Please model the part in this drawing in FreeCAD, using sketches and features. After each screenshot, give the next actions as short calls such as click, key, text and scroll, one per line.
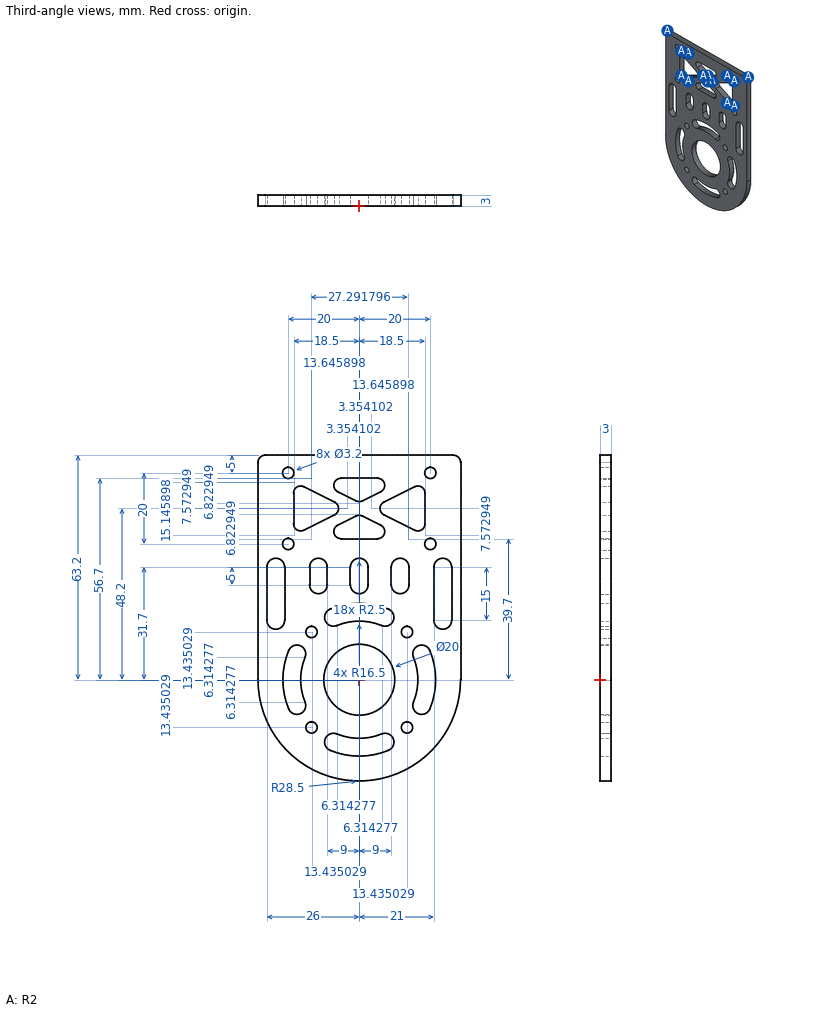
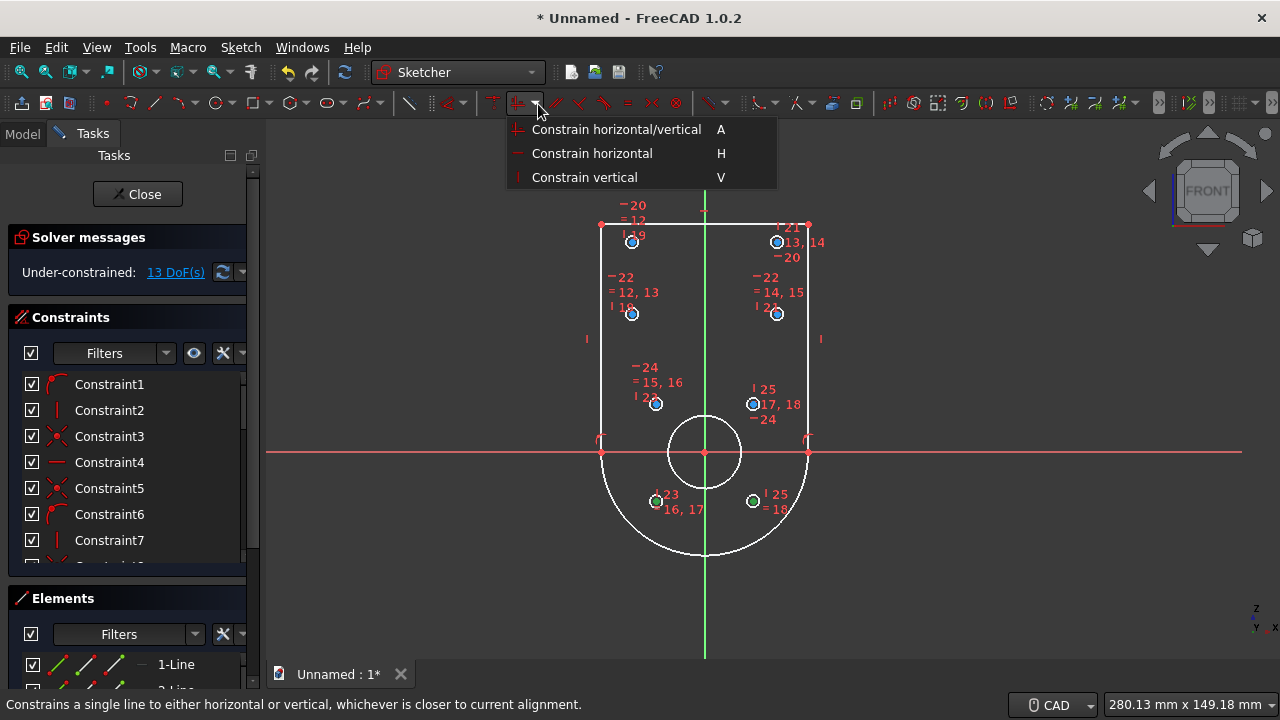
click(642, 153)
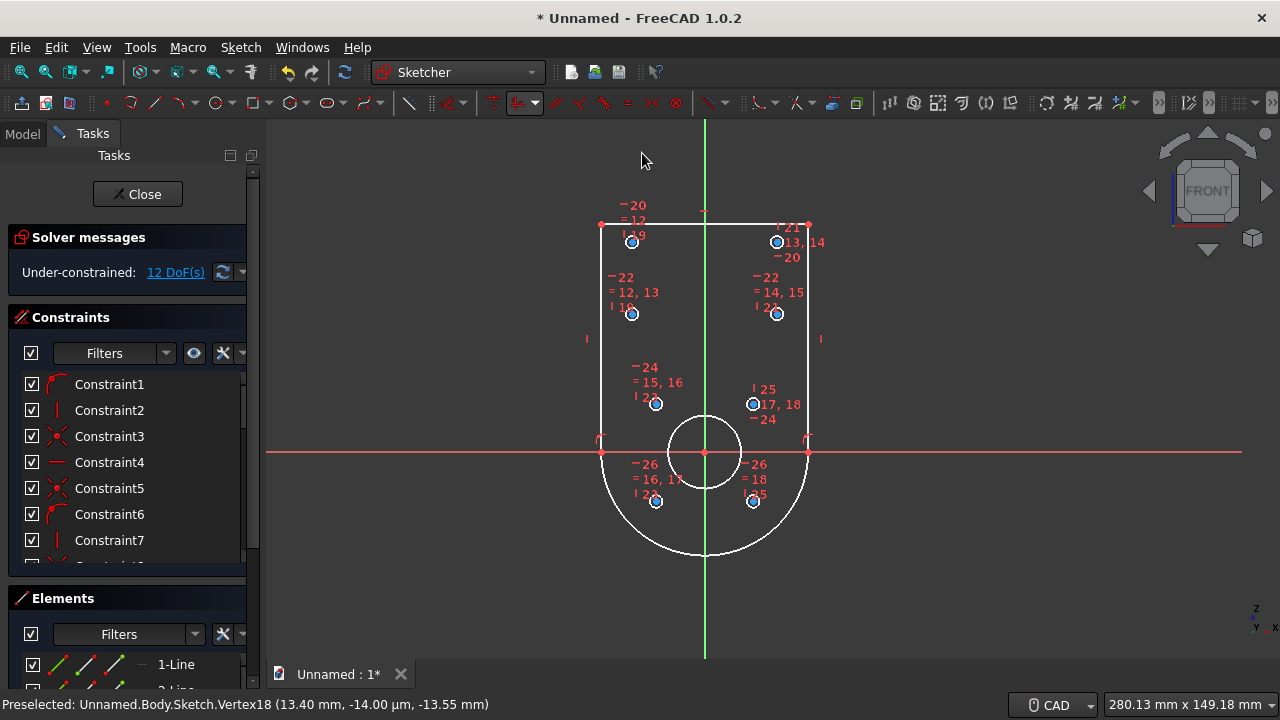
key(d)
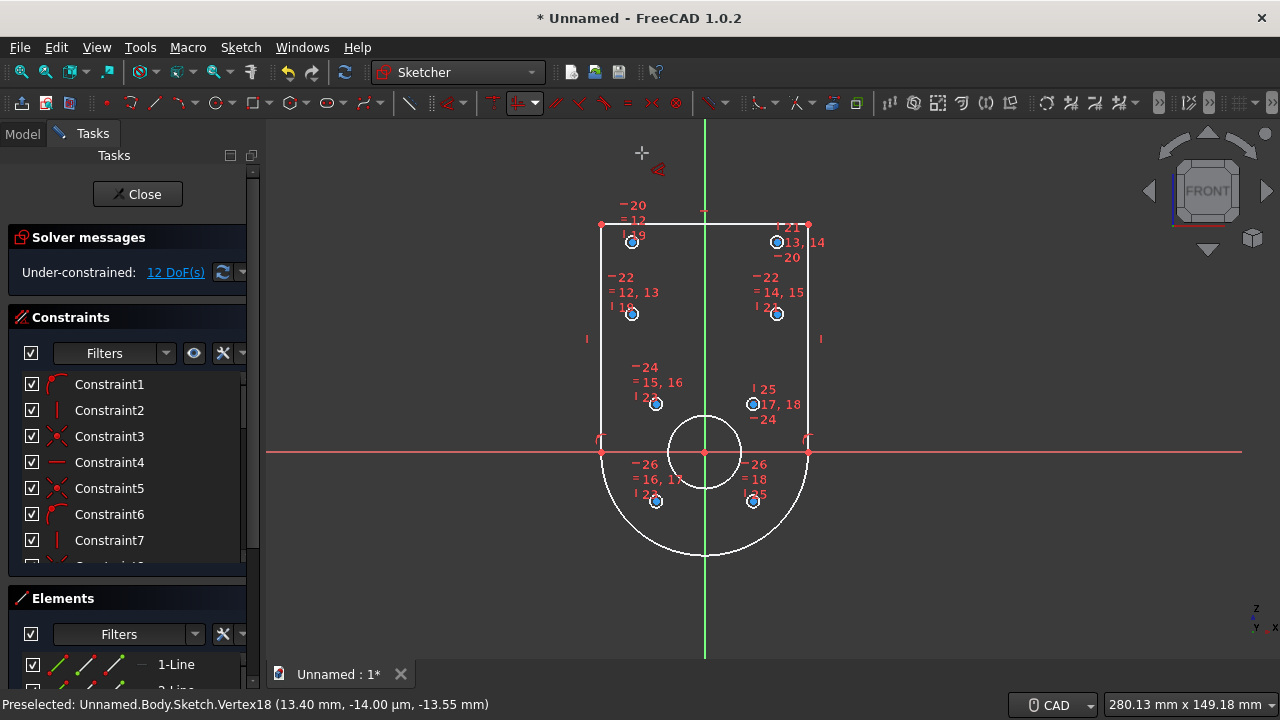
click(644, 536)
click(625, 562)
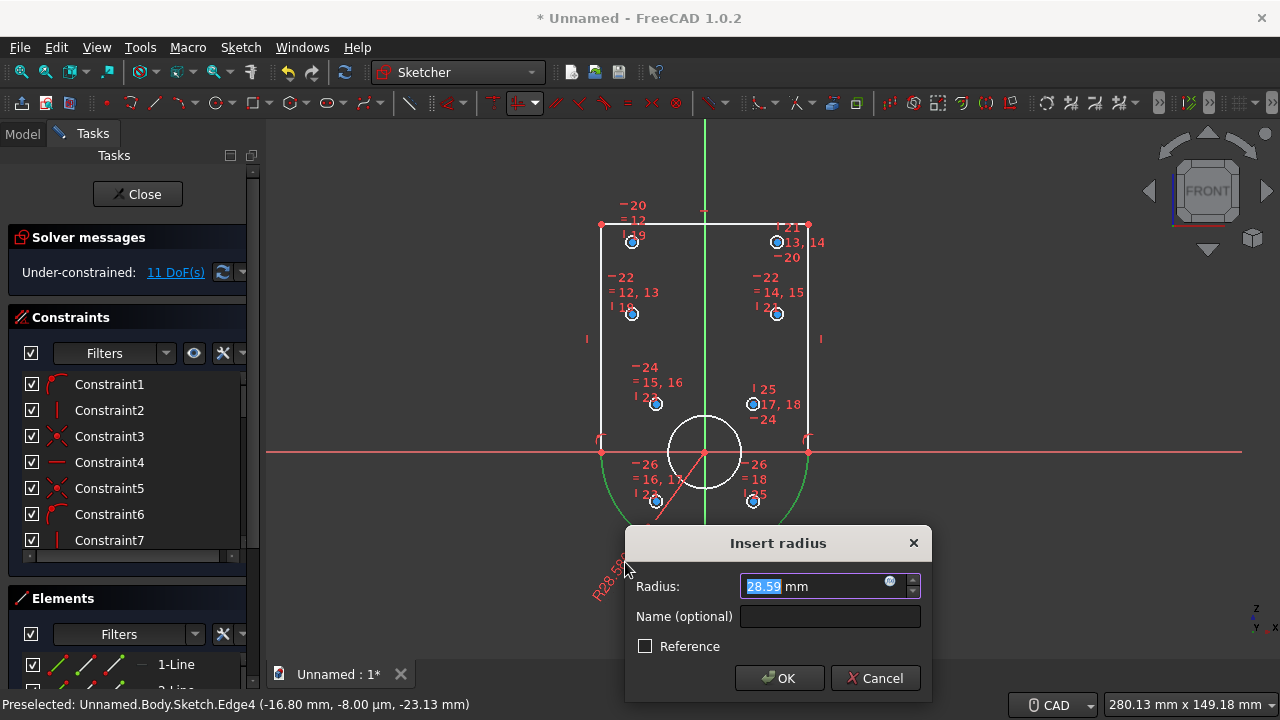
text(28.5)
key(Return)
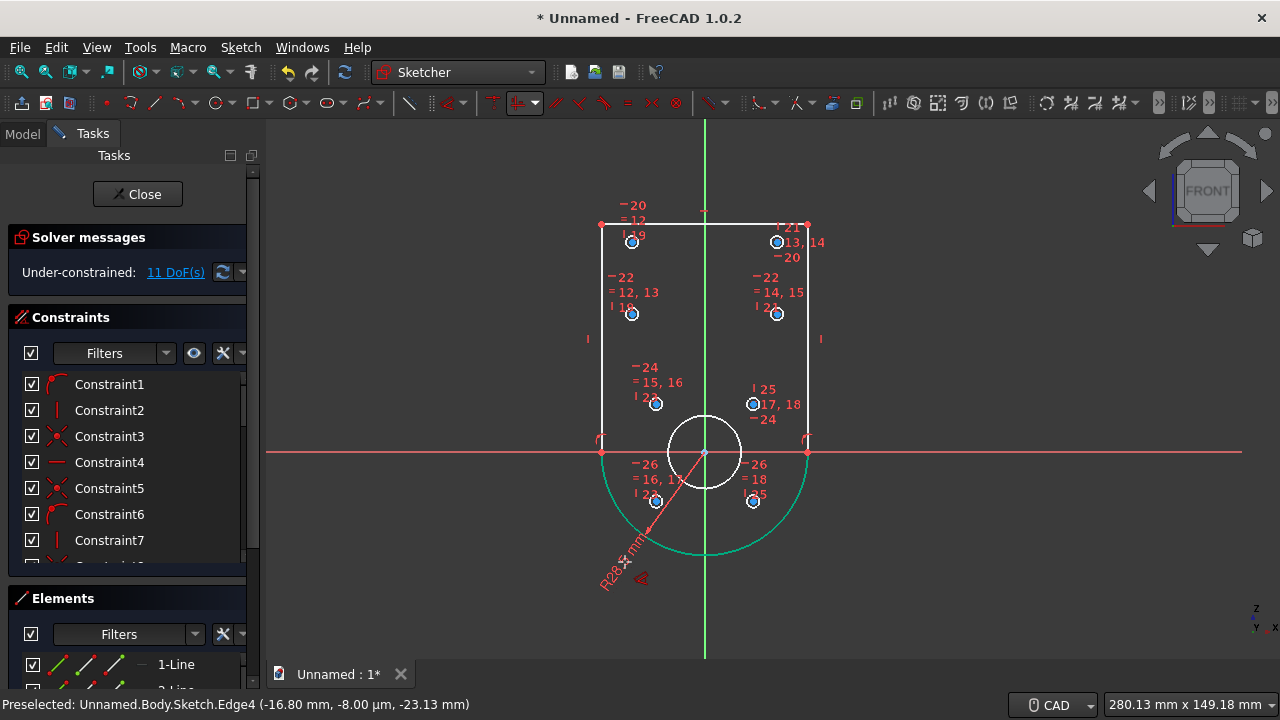
scroll(632, 248, up, 7)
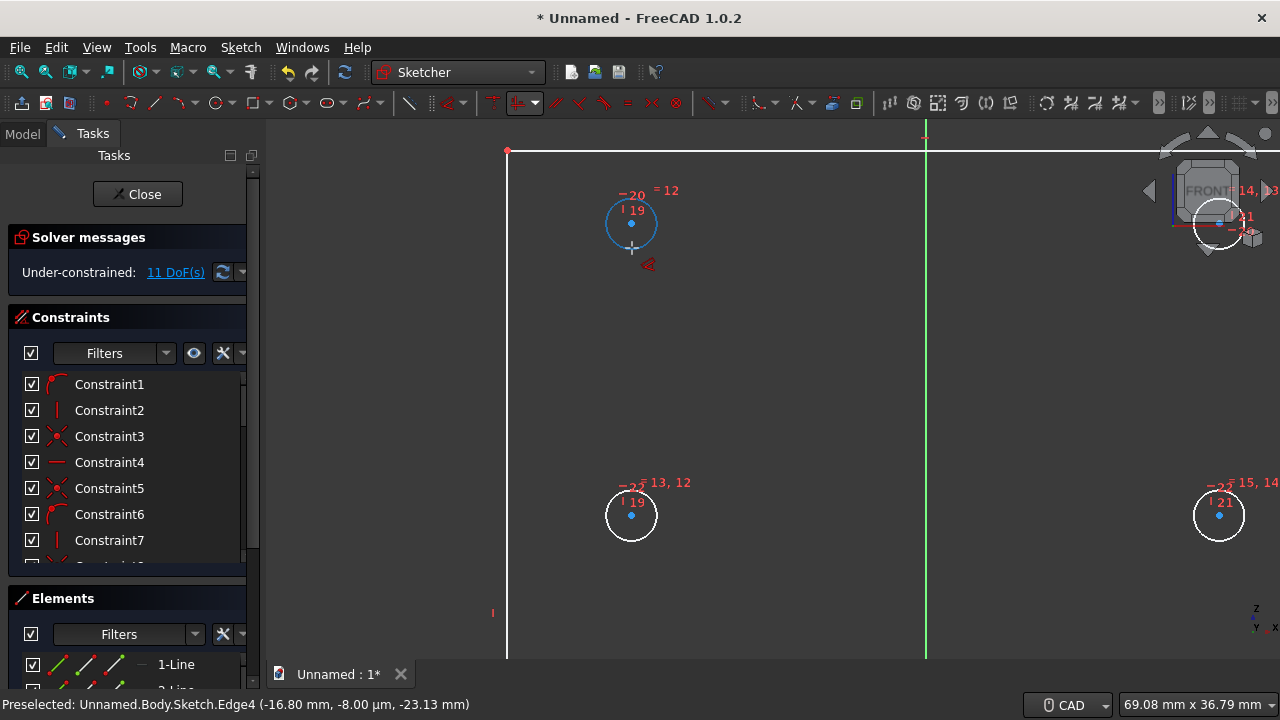
click(631, 249)
click(630, 281)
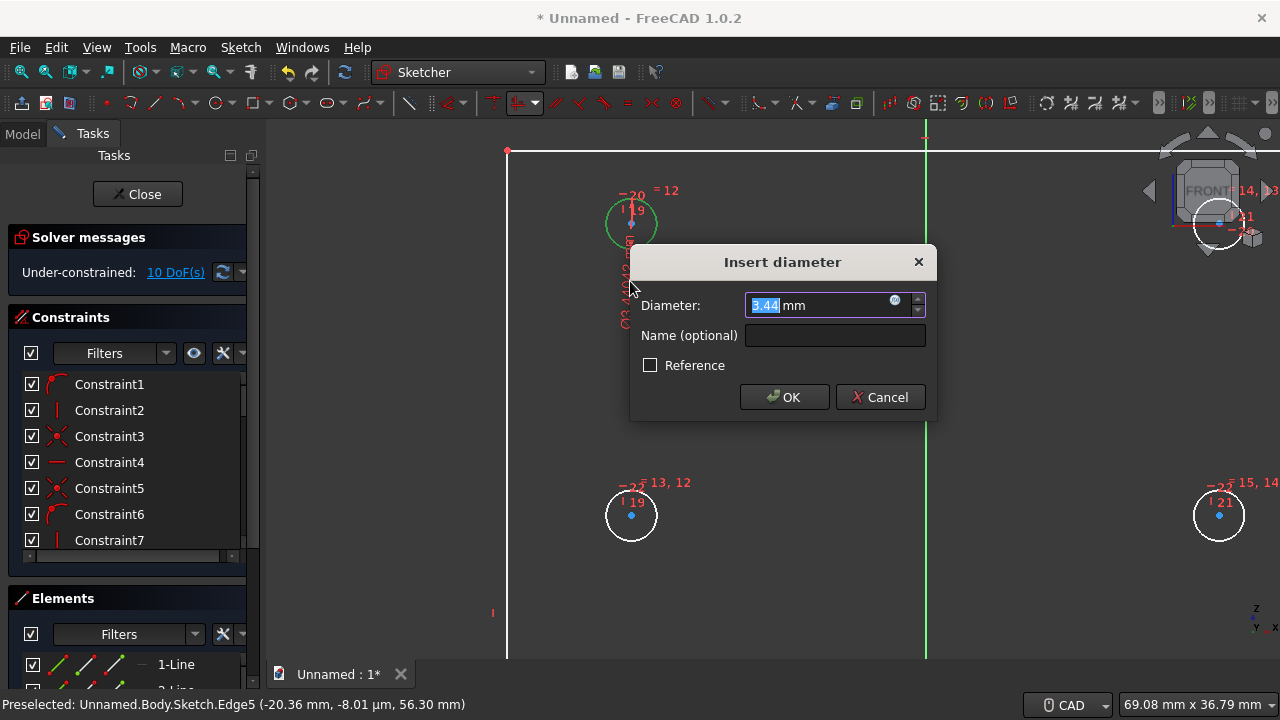
text(3.2)
key(Return)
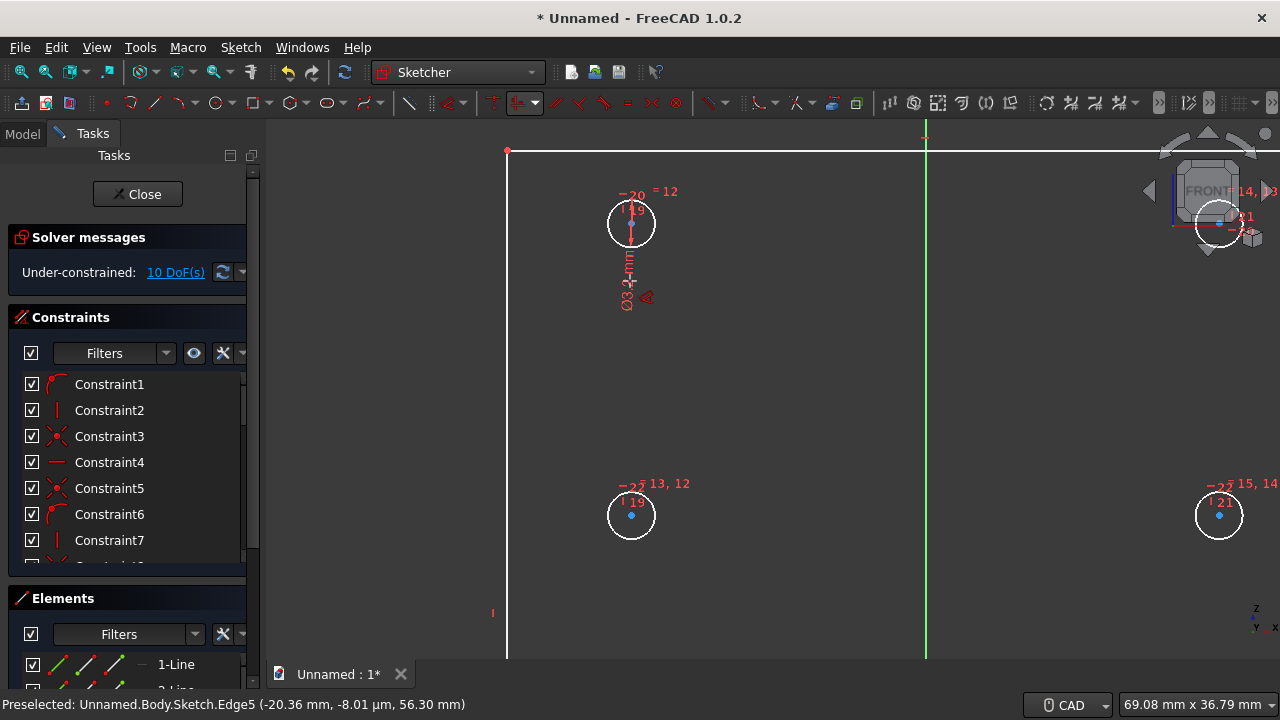
scroll(632, 248, down, 7)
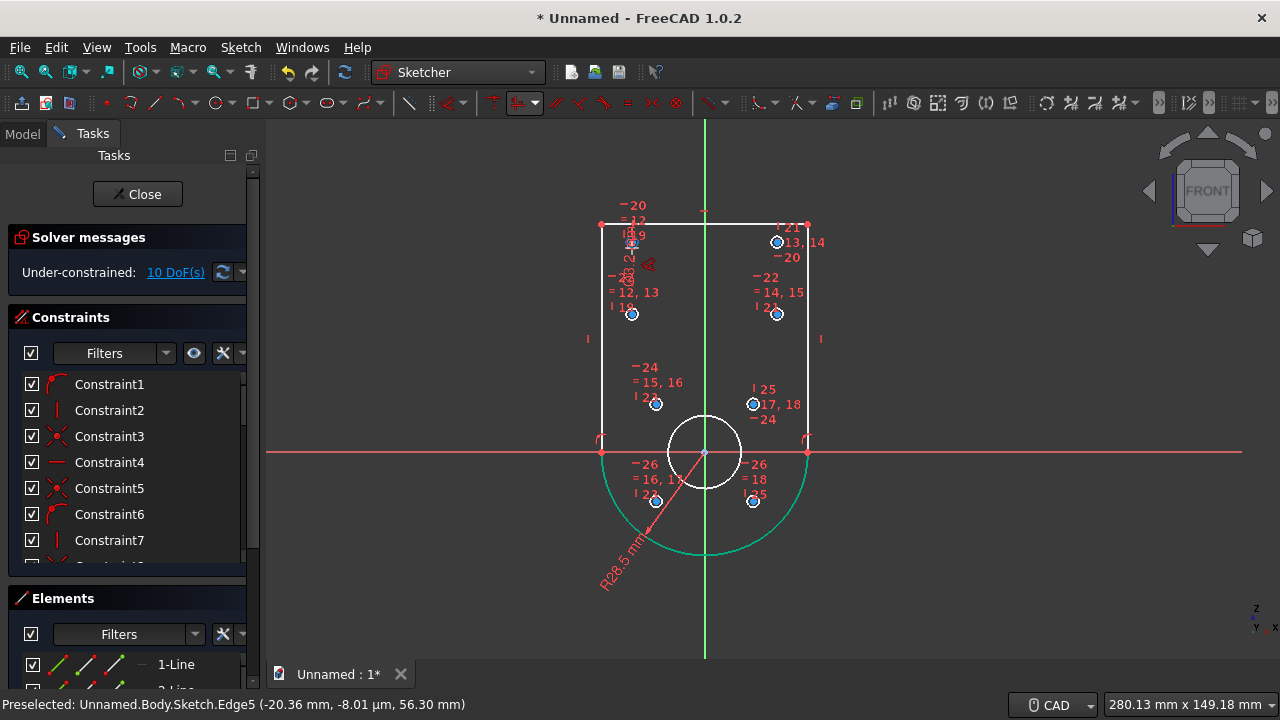
click(730, 426)
click(770, 432)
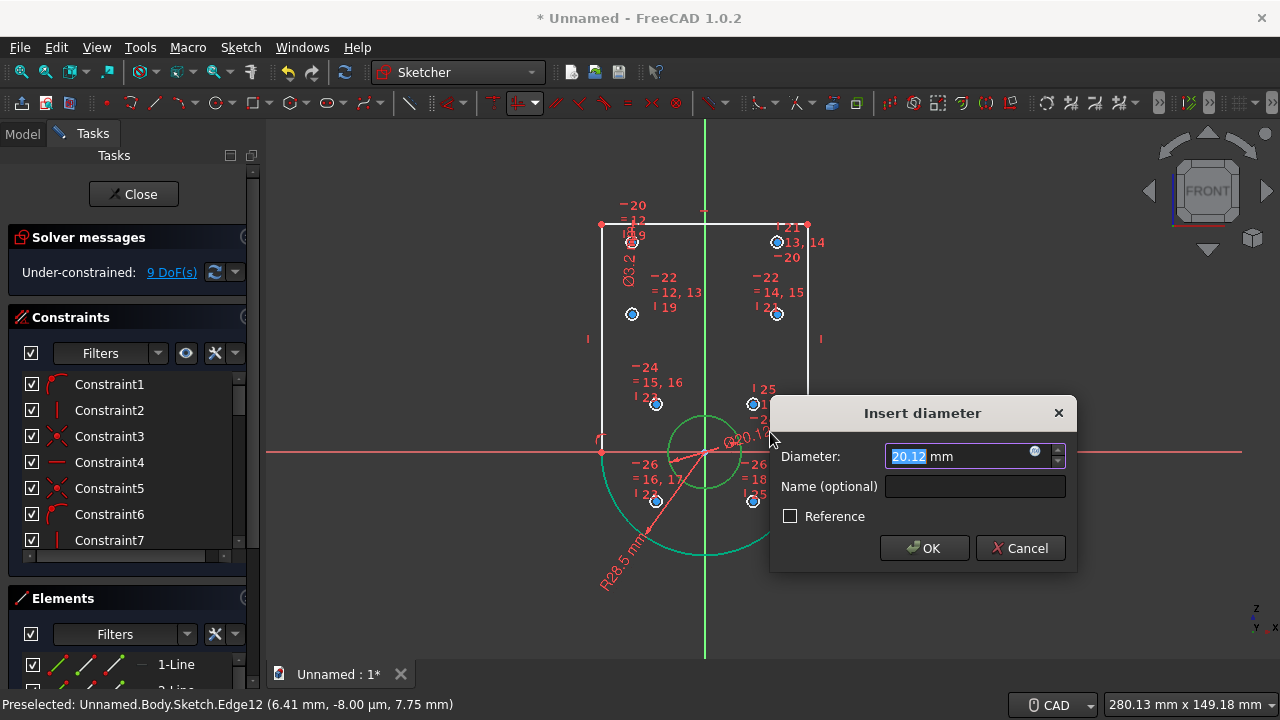
text(20)
key(Return)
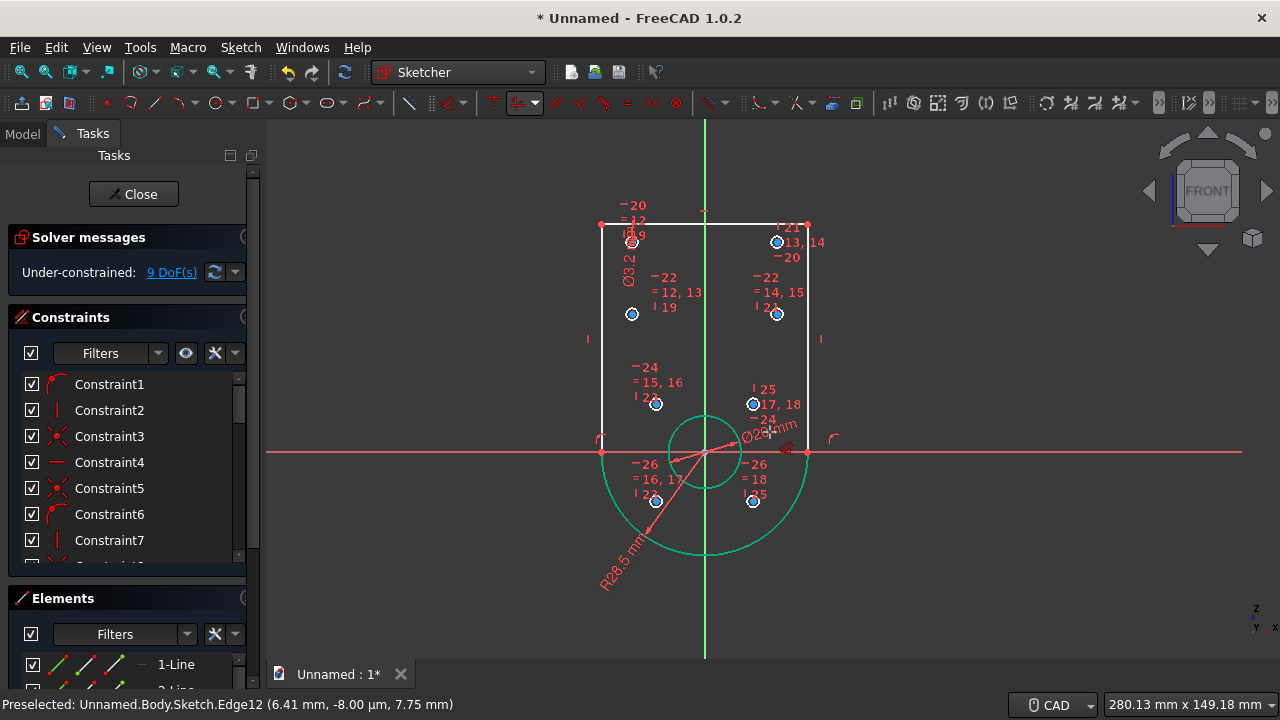
click(632, 242)
click(668, 208)